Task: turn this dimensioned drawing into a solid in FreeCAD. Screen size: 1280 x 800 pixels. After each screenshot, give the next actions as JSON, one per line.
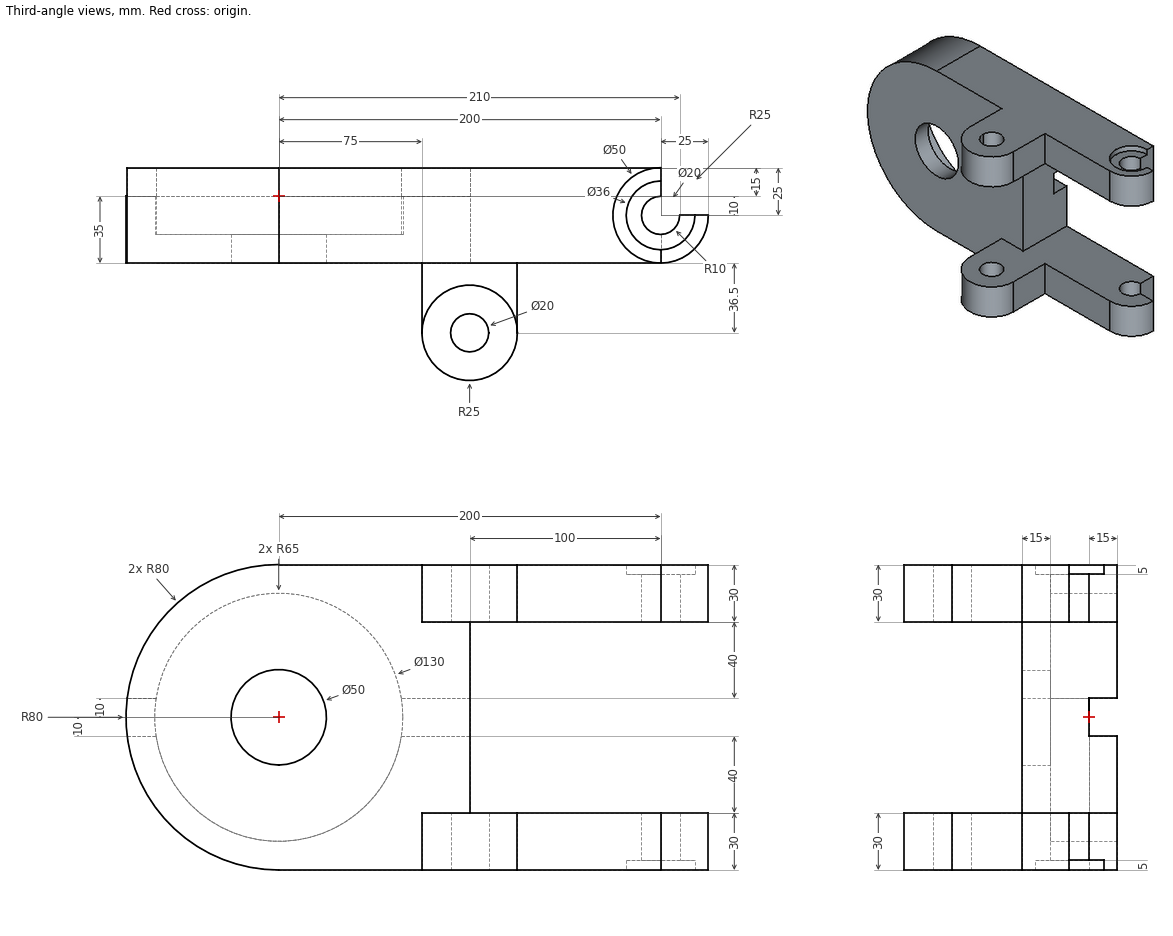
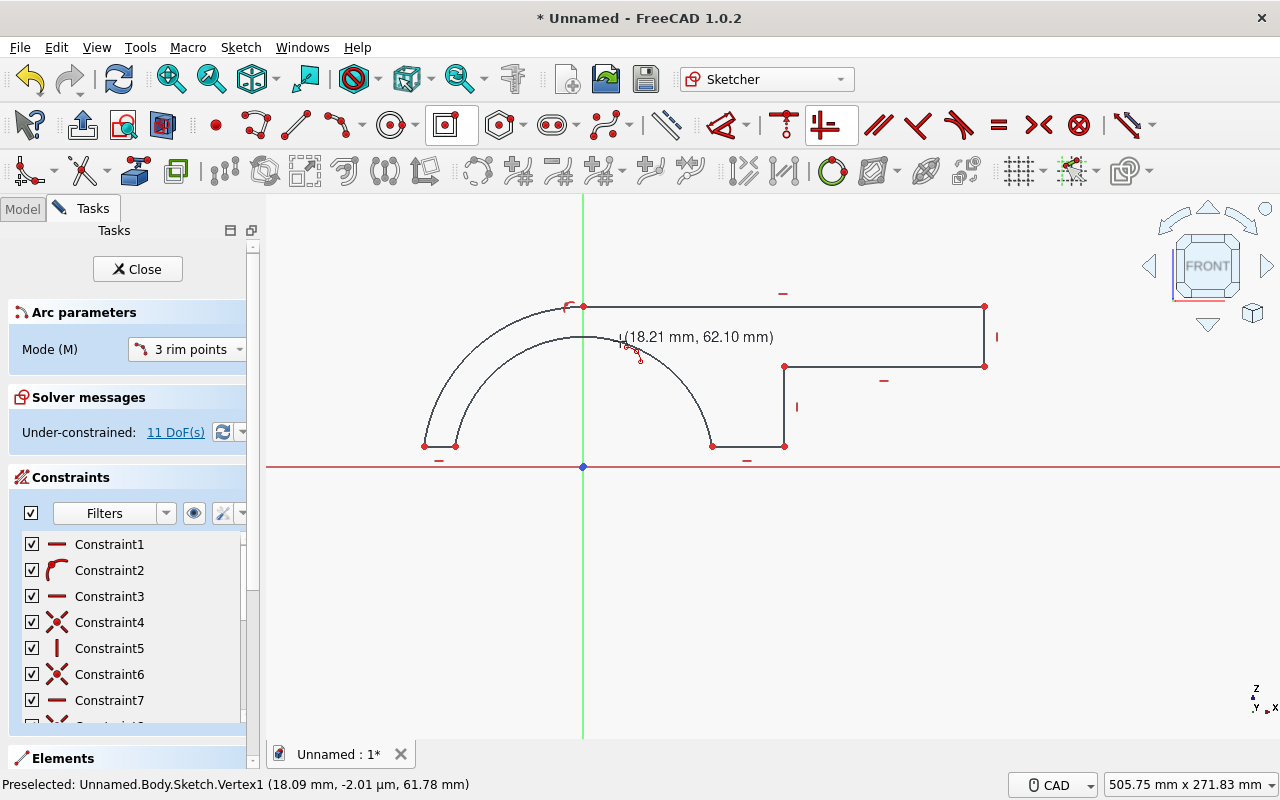
{"action": "left_click", "coordinate": [296, 126]}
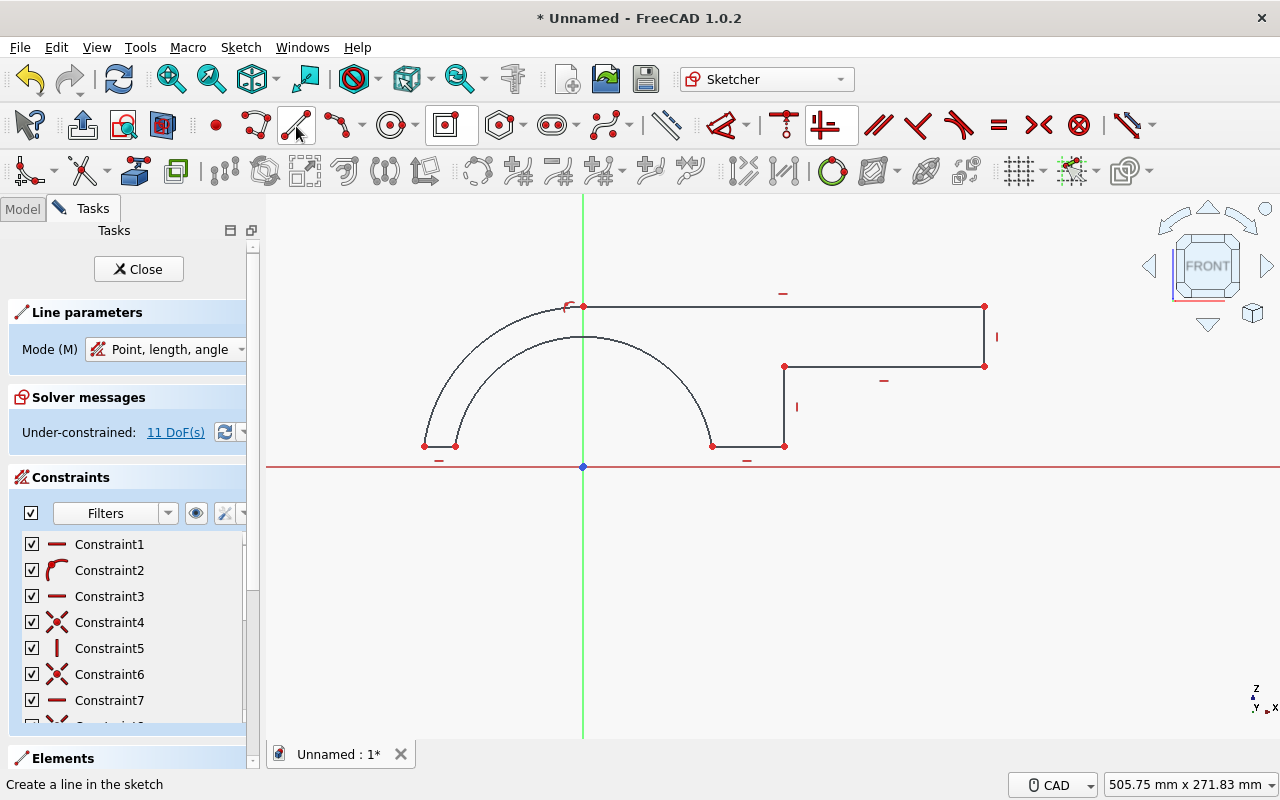
{"action": "left_click", "coordinate": [424, 487]}
{"action": "left_click", "coordinate": [455, 487]}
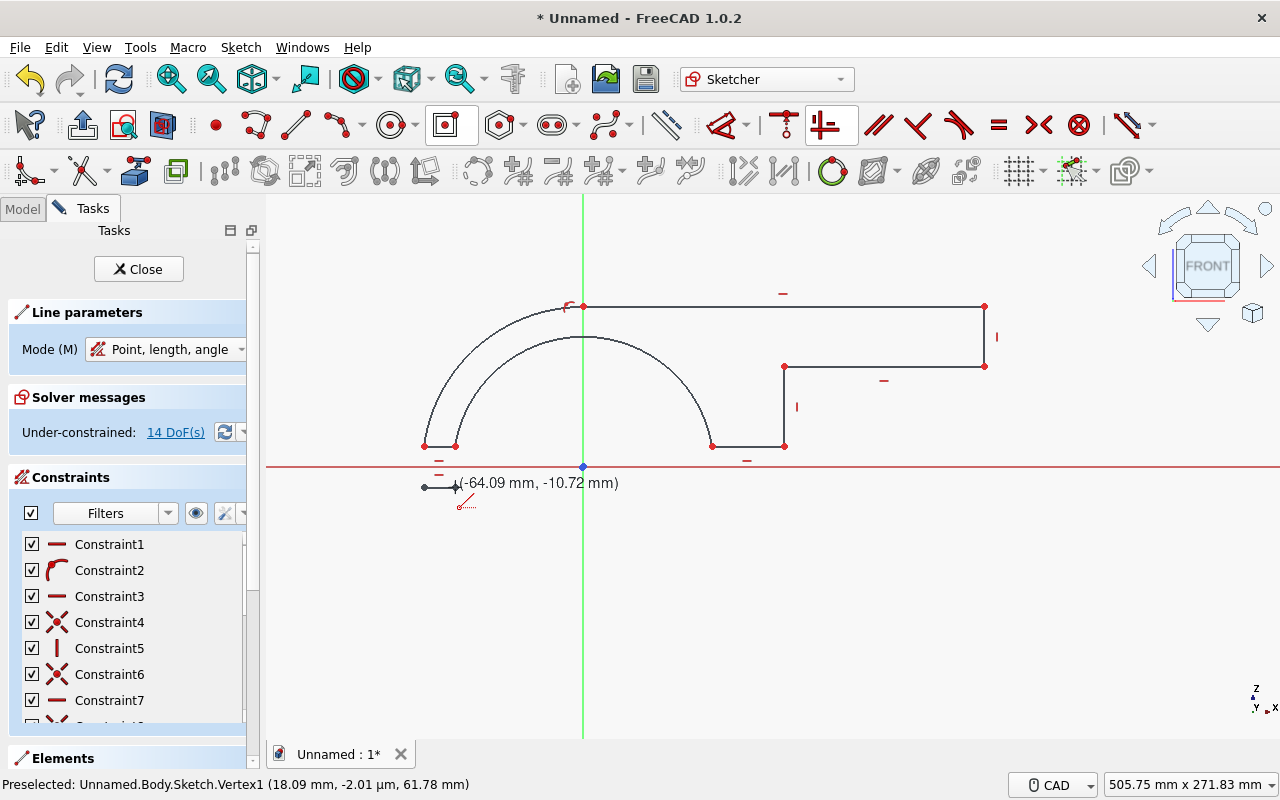
{"action": "left_click", "coordinate": [256, 126]}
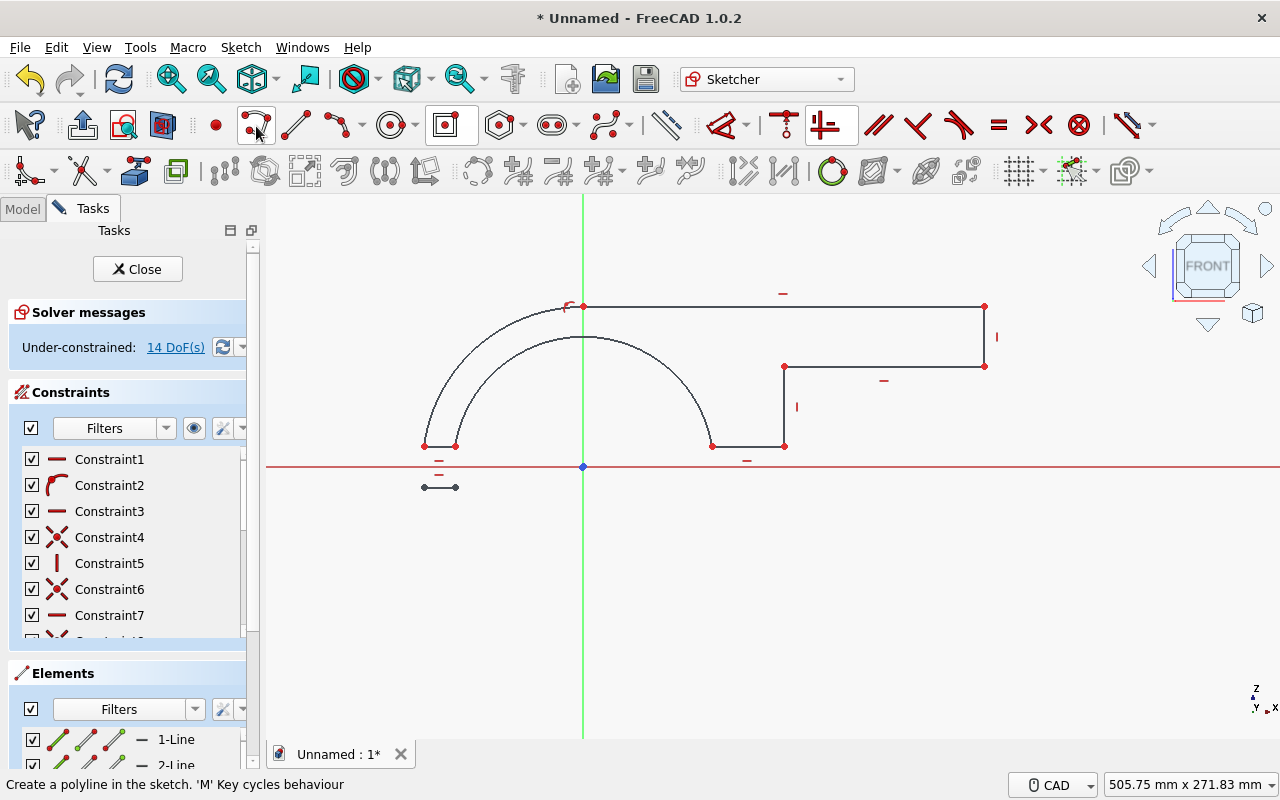
{"action": "left_click", "coordinate": [712, 487]}
{"action": "left_click", "coordinate": [784, 487]}
{"action": "left_click", "coordinate": [784, 567]}
{"action": "left_click", "coordinate": [984, 567]}
{"action": "left_click", "coordinate": [984, 627]}
{"action": "left_click", "coordinate": [583, 627]}
{"action": "right_click", "coordinate": [583, 627]}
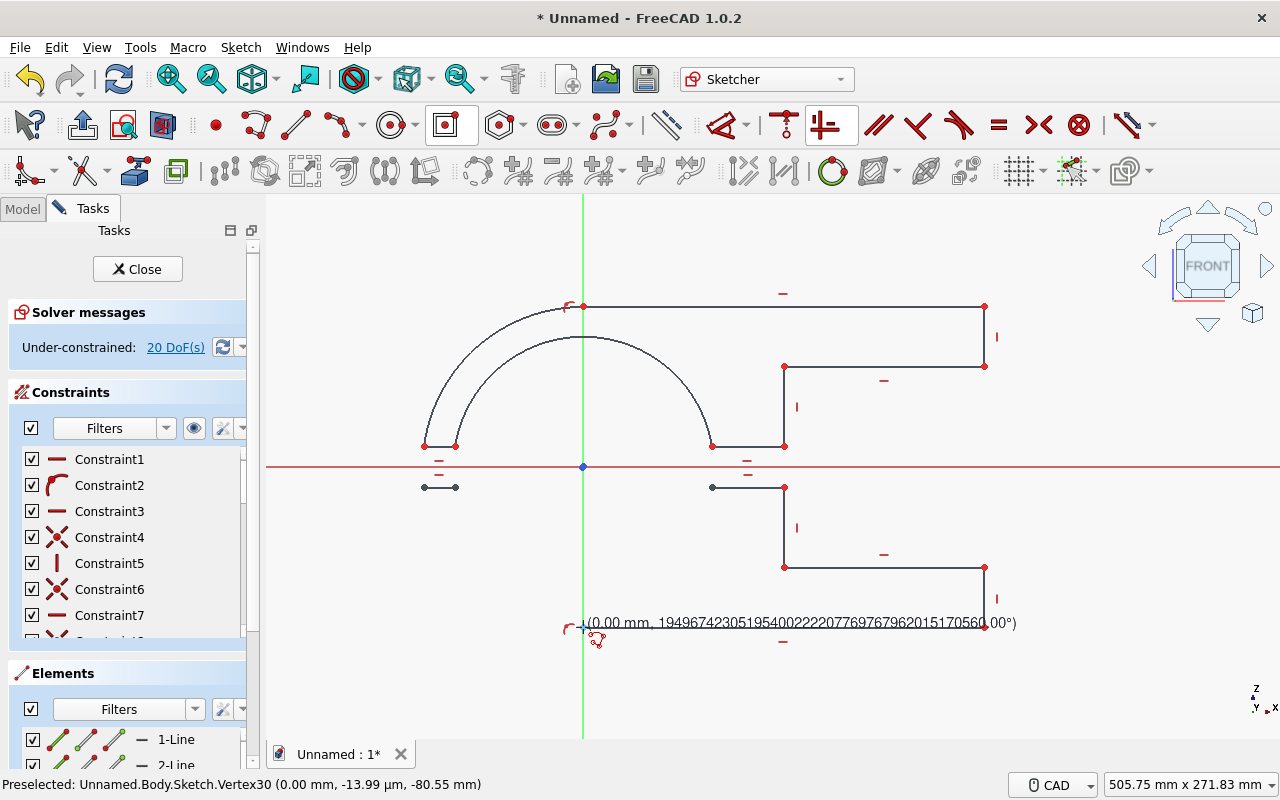
{"action": "left_click", "coordinate": [338, 126]}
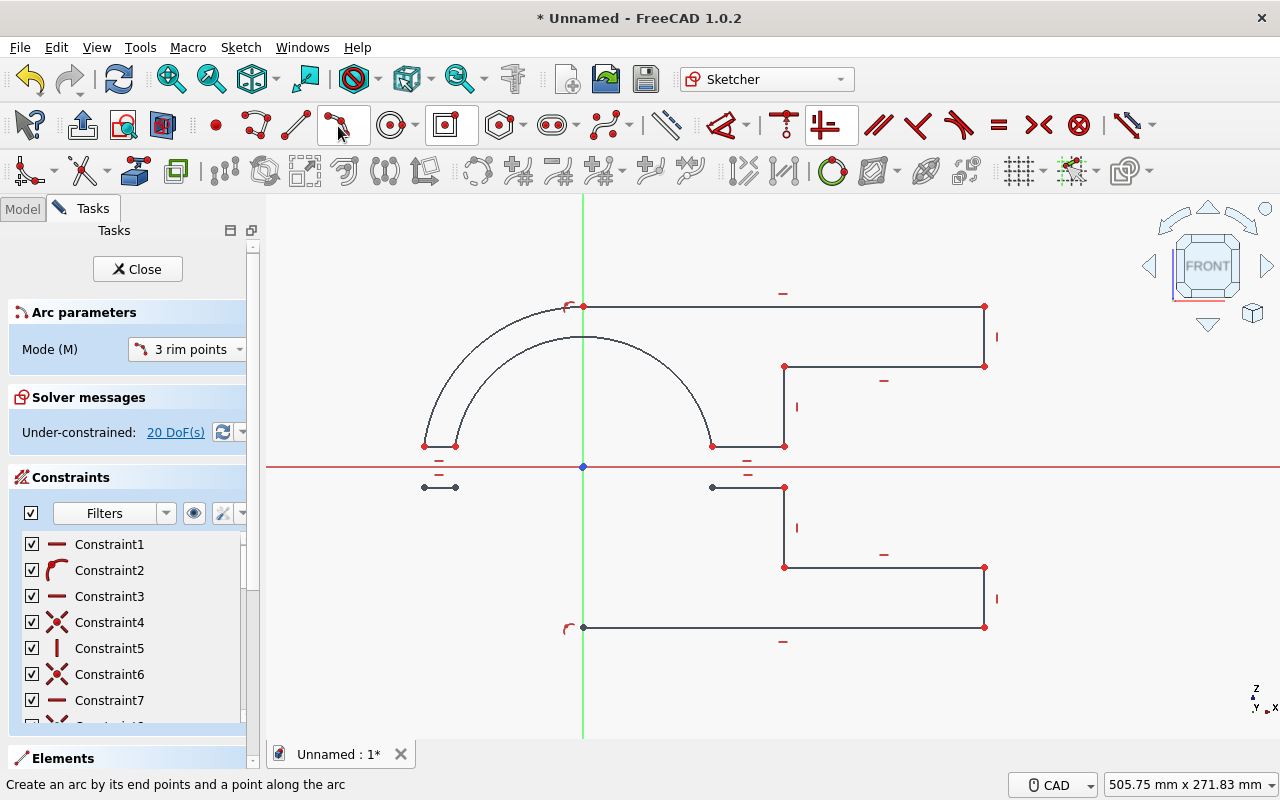
{"action": "left_click", "coordinate": [455, 488]}
{"action": "left_click", "coordinate": [712, 488]}
{"action": "left_click", "coordinate": [547, 592]}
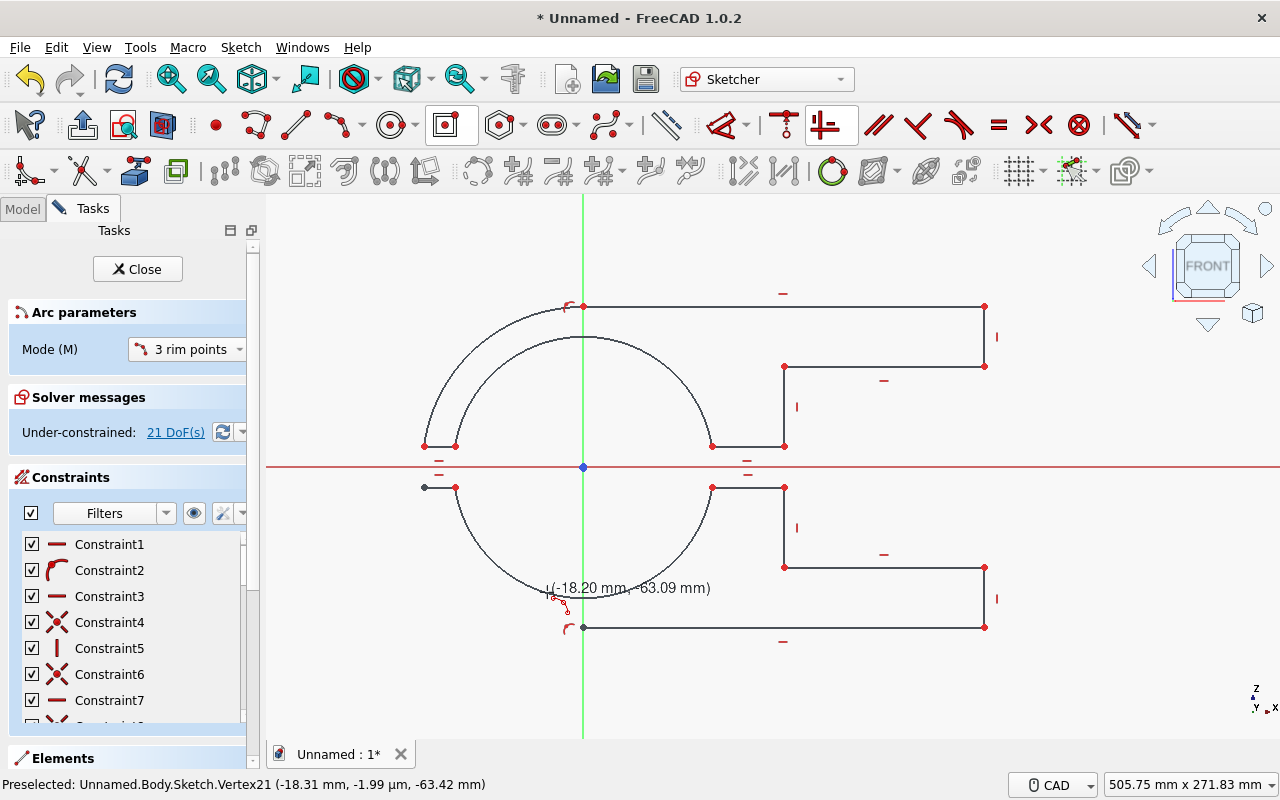
{"action": "left_click", "coordinate": [583, 628]}
{"action": "left_click", "coordinate": [424, 488]}
{"action": "left_click", "coordinate": [477, 587]}
{"action": "key", "text": "Escape"}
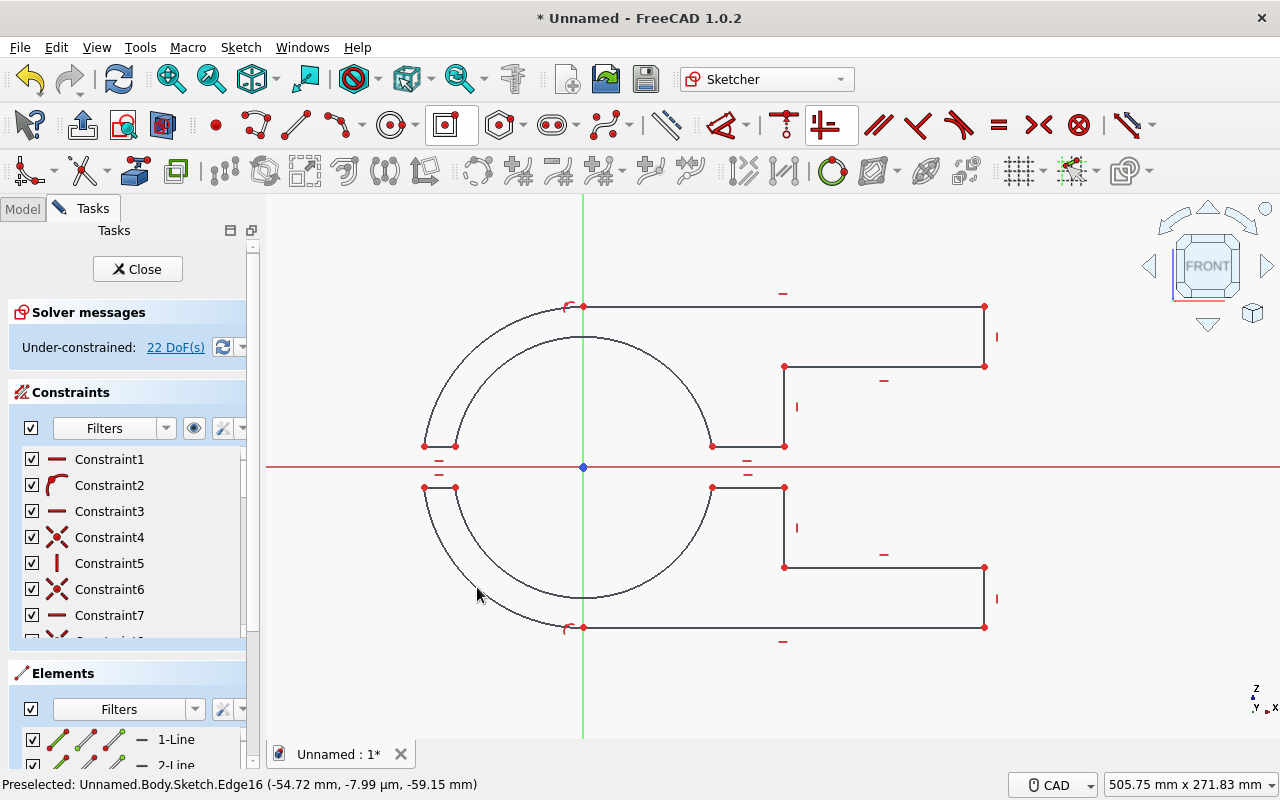
{"action": "left_click", "coordinate": [516, 322]}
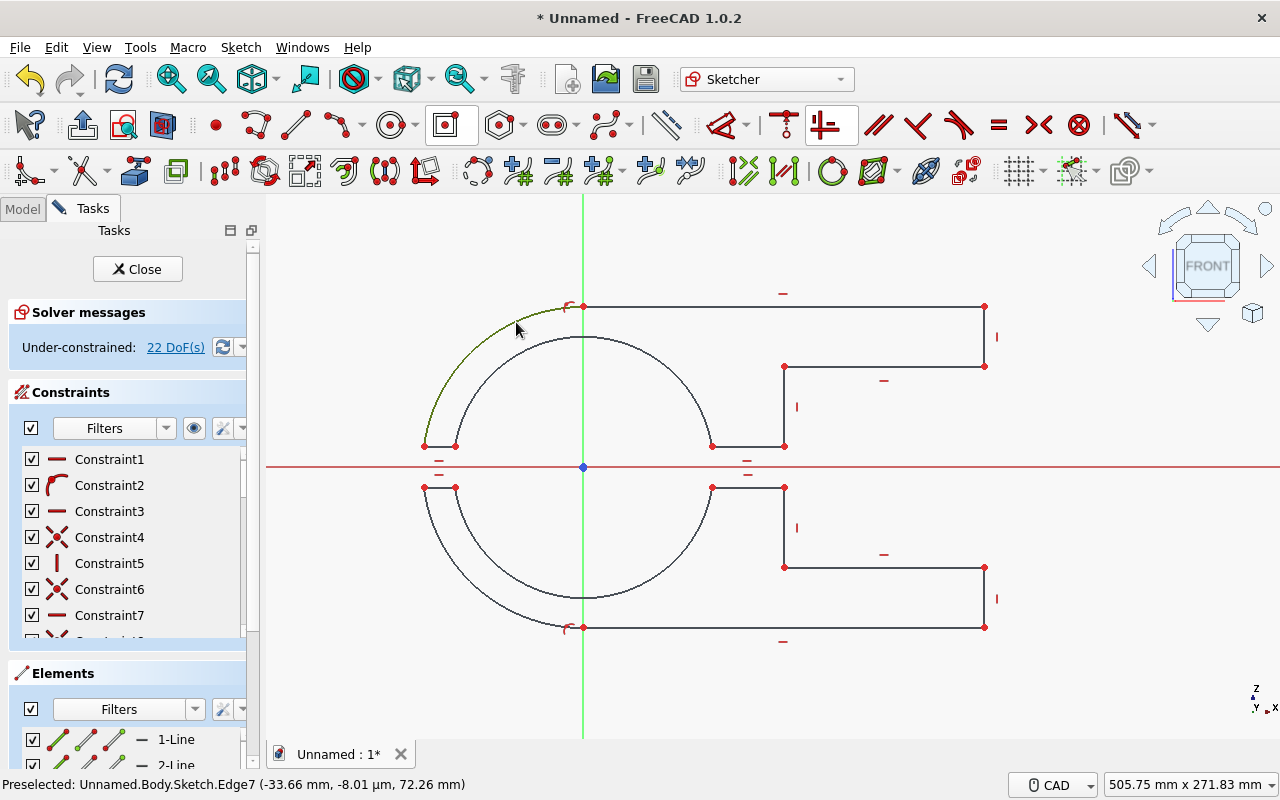
{"action": "left_click", "coordinate": [653, 357]}